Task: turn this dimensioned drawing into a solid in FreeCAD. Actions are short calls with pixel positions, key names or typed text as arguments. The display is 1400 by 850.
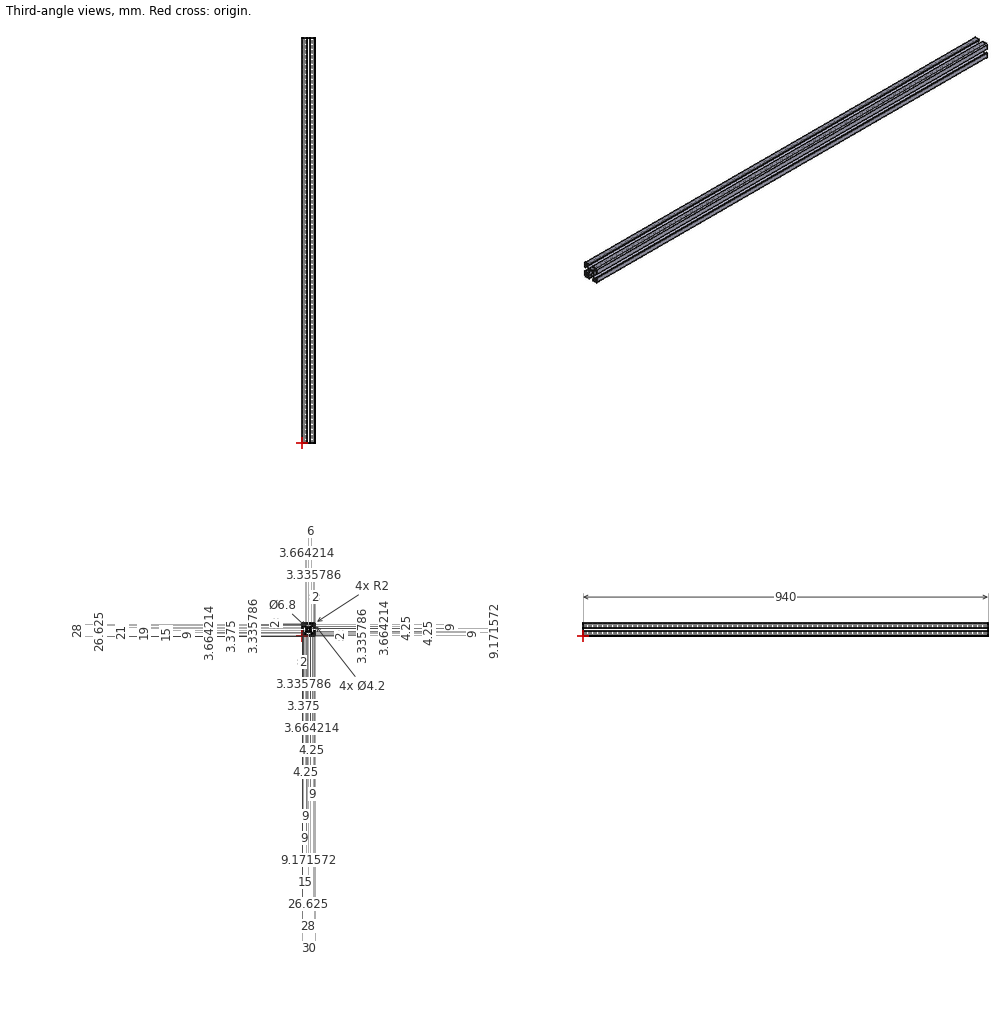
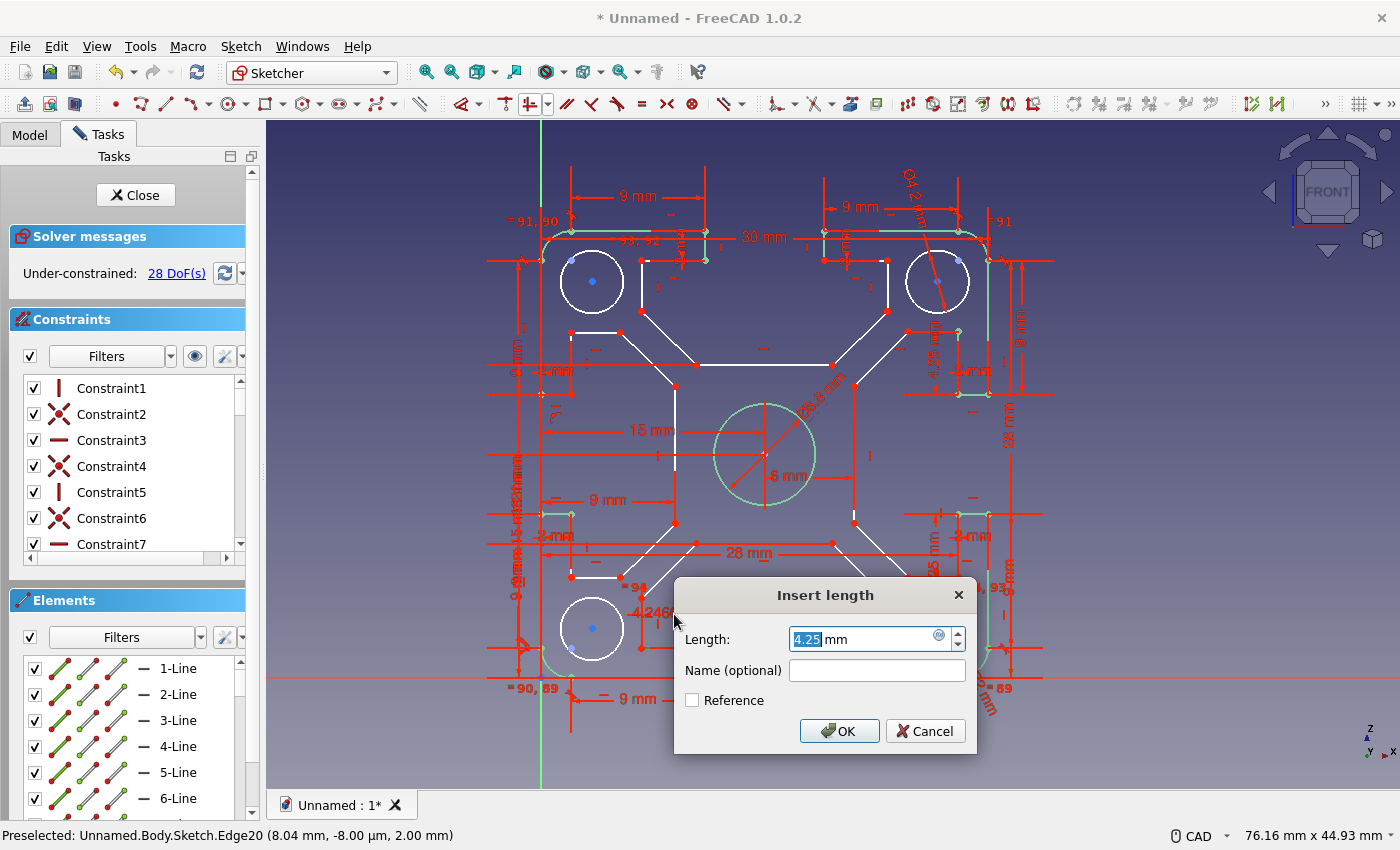
text(4.25)
key(Return)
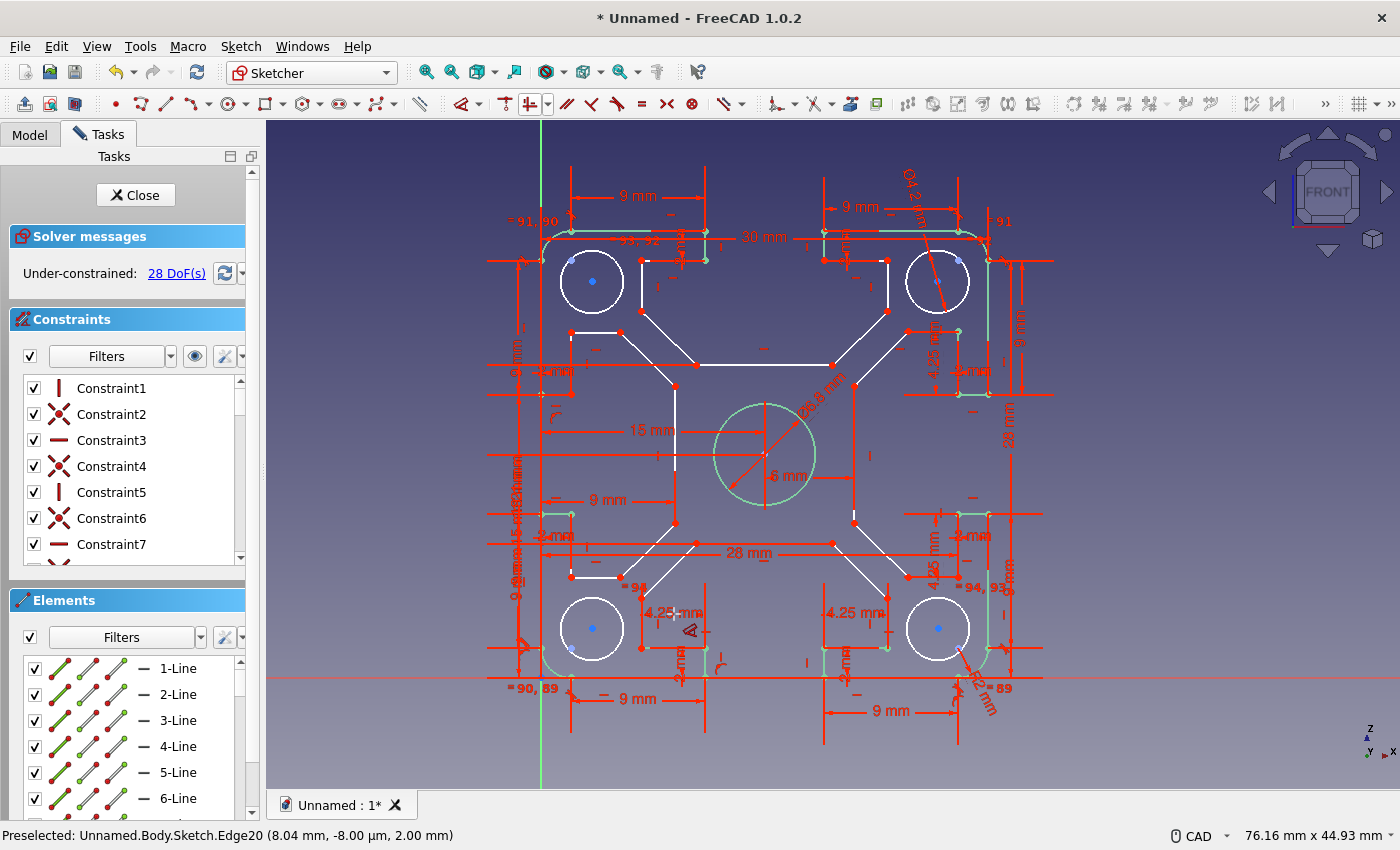
click(571, 533)
click(605, 561)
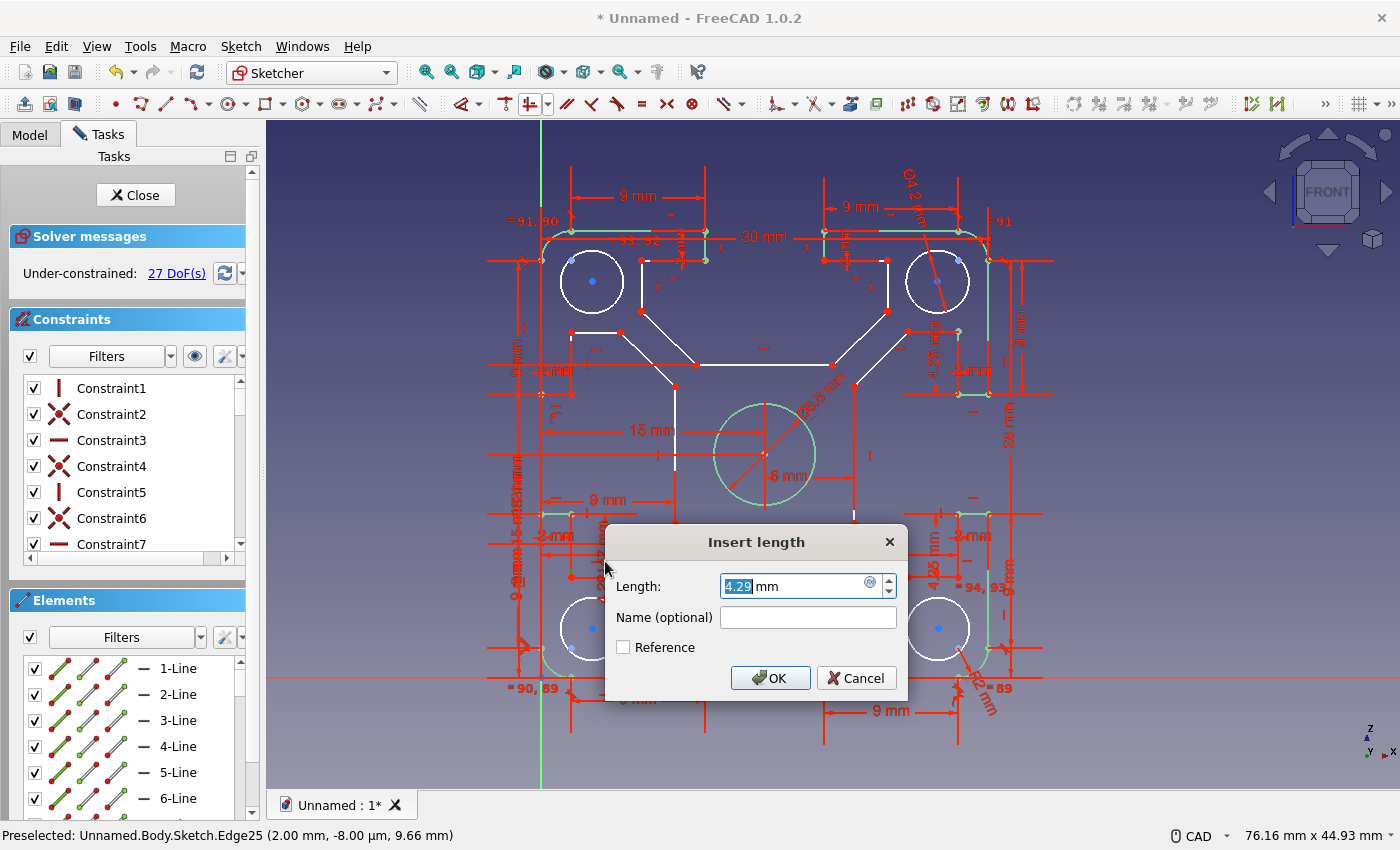
text(4.25)
key(Return)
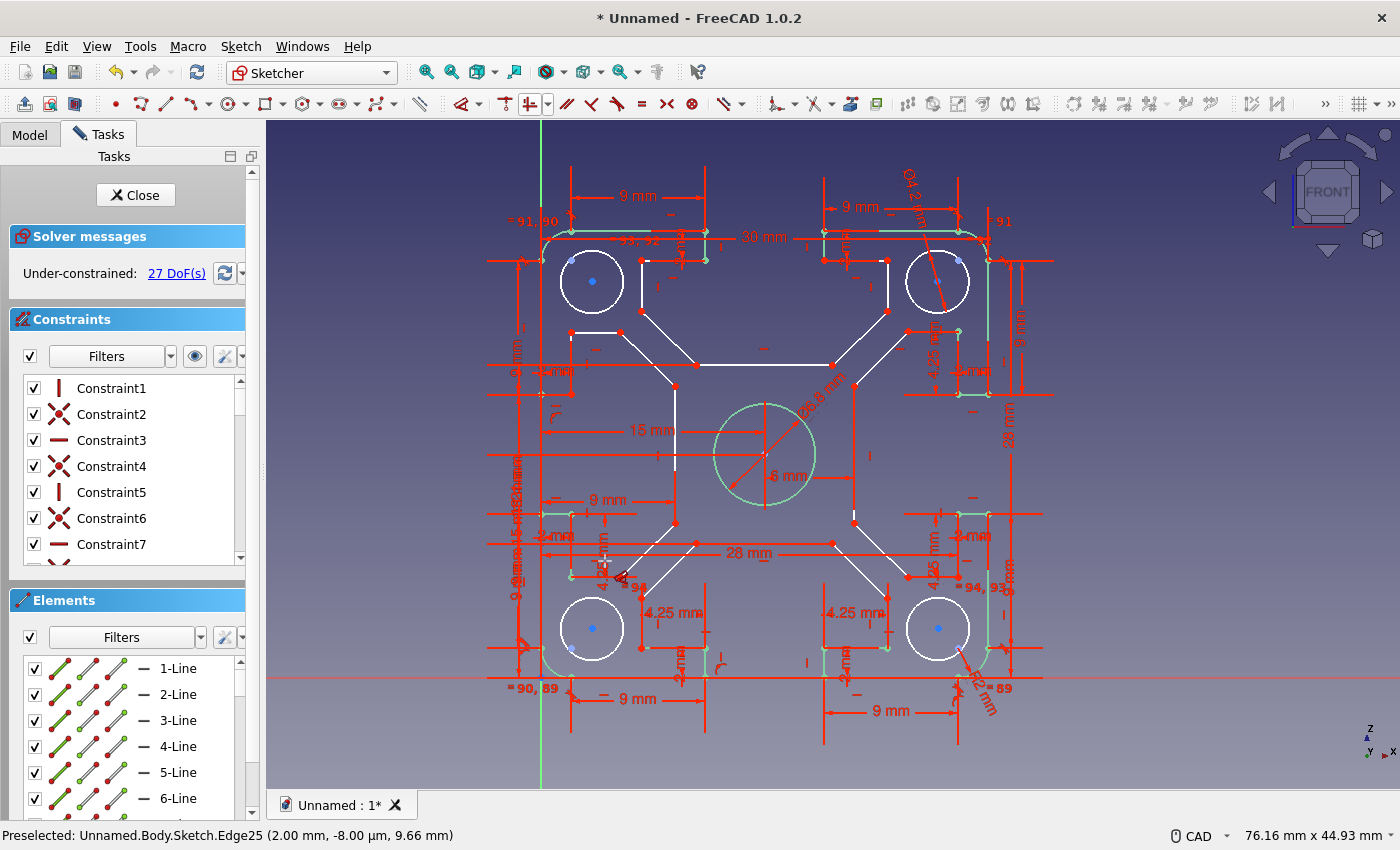
click(571, 352)
click(605, 350)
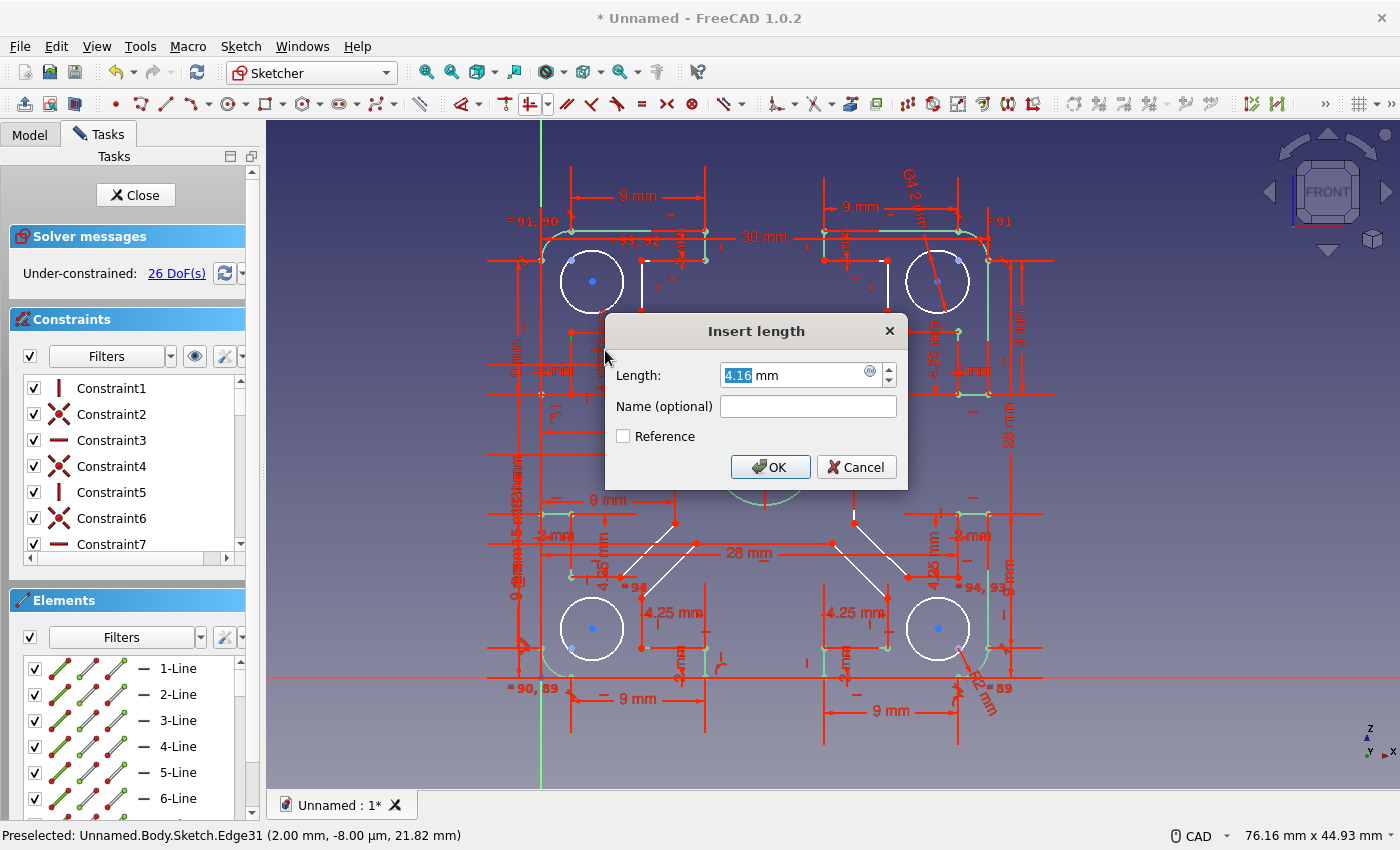
text(4.25)
key(Return)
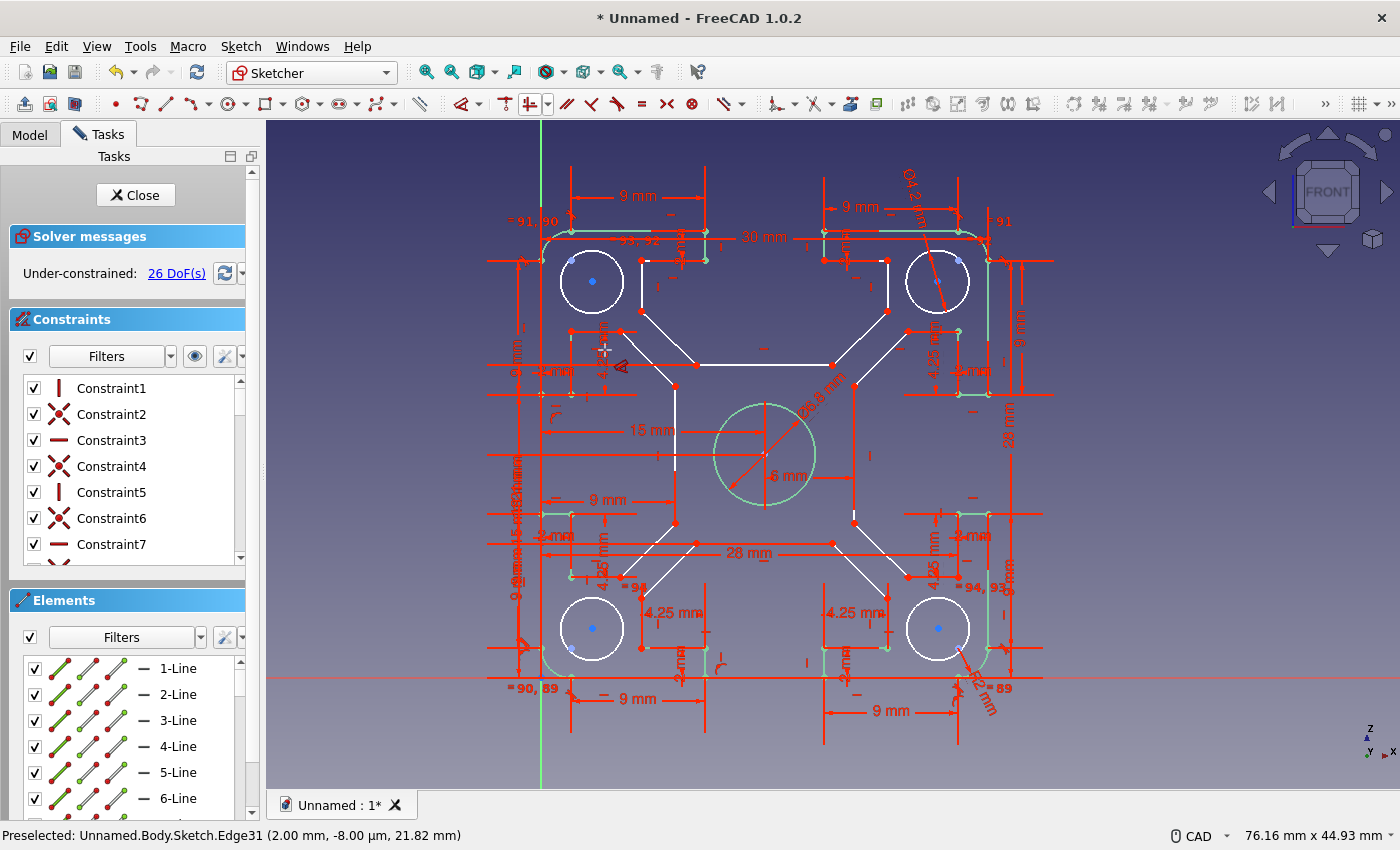
click(686, 261)
click(674, 295)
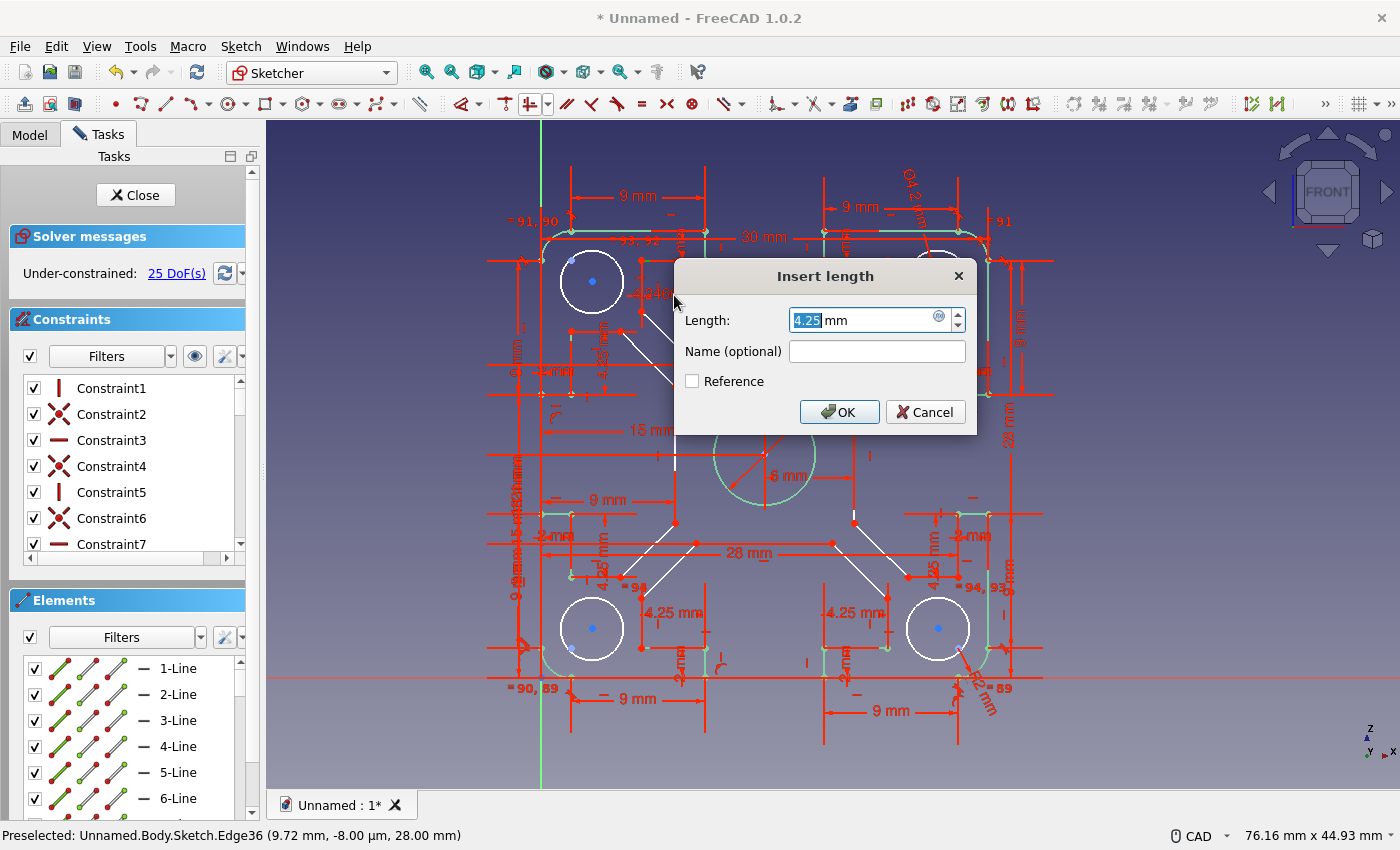
text(4.25)
key(Return)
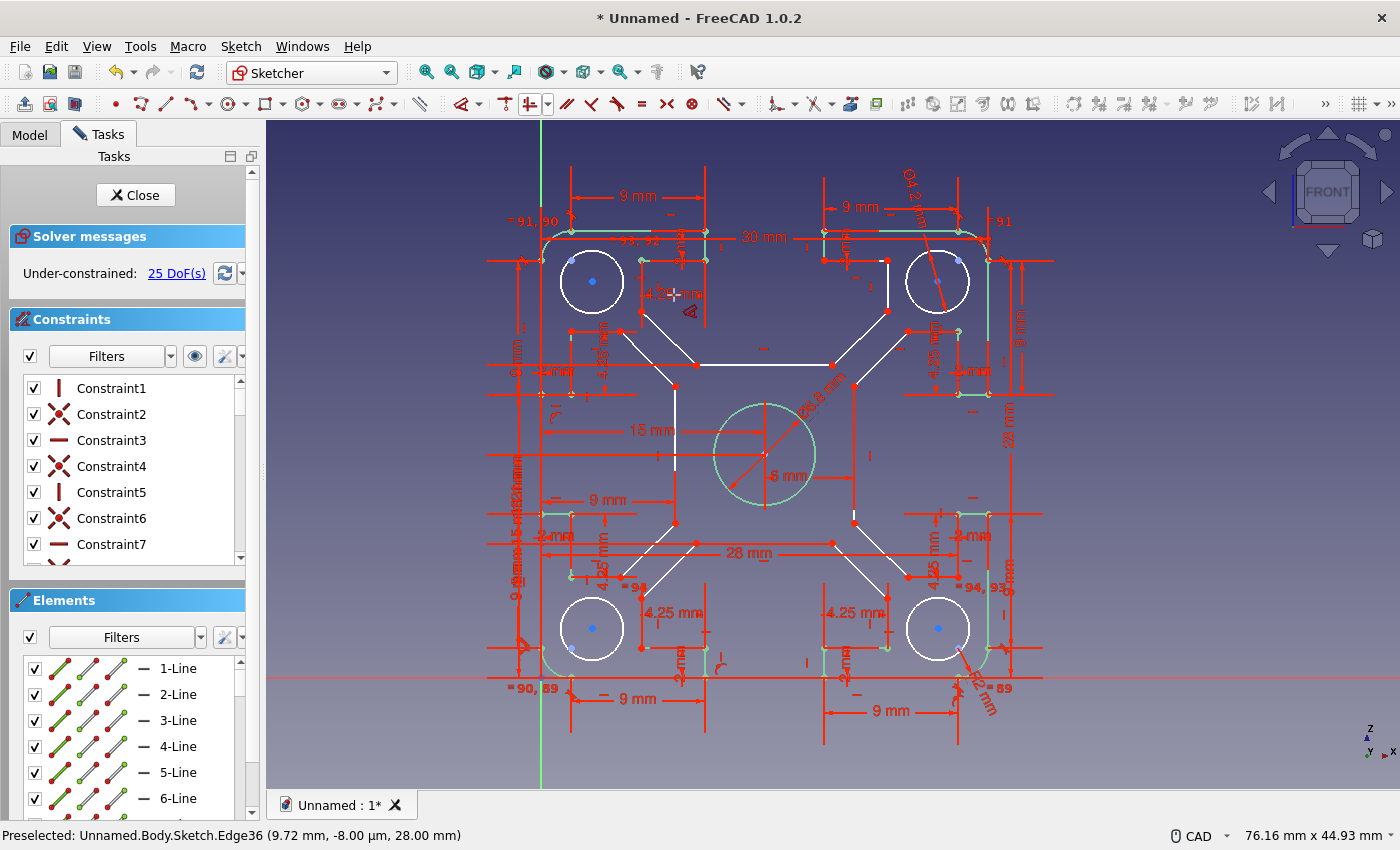
click(869, 261)
click(856, 295)